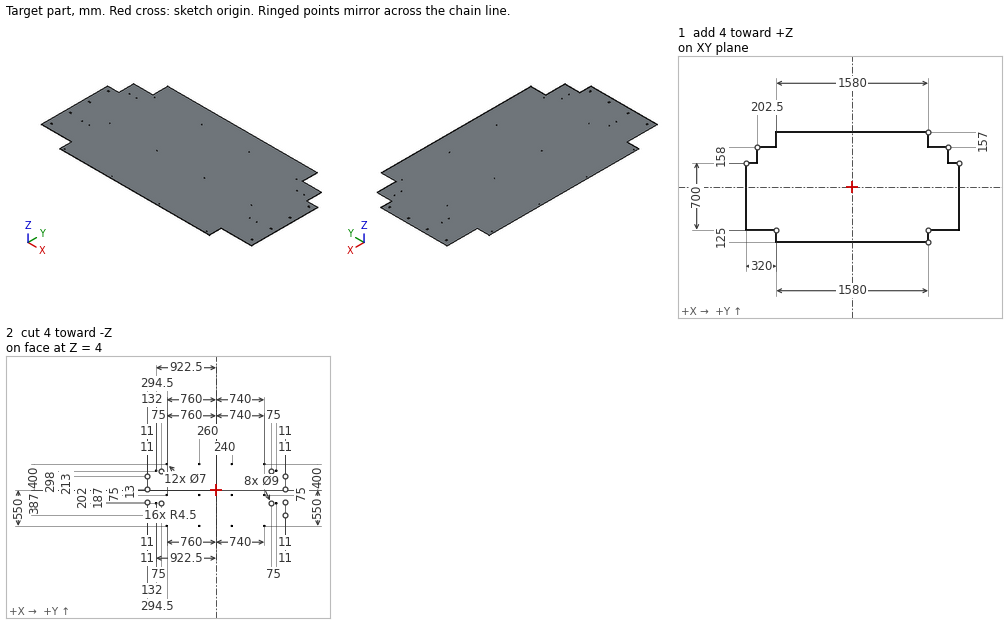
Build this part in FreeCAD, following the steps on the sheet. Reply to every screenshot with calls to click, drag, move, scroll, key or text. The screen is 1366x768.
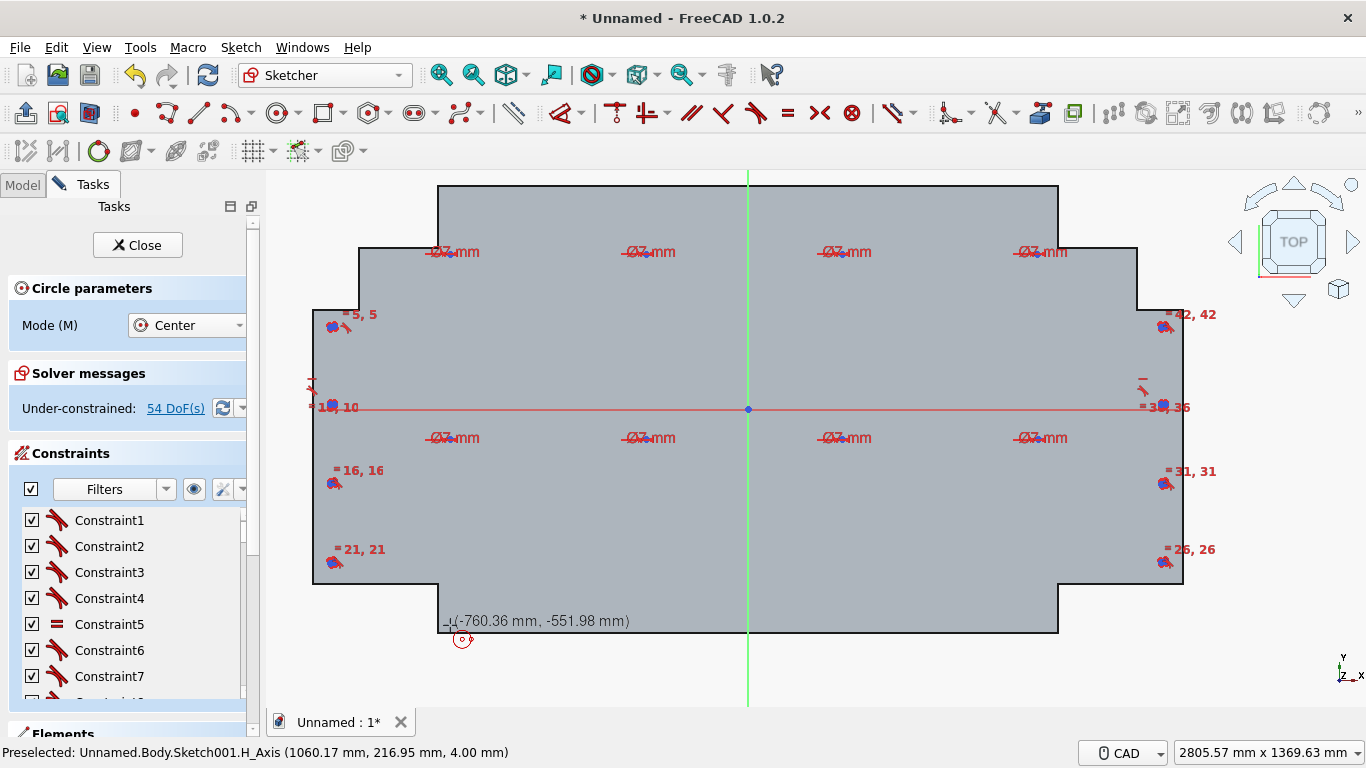
click(450, 625)
move(451, 624)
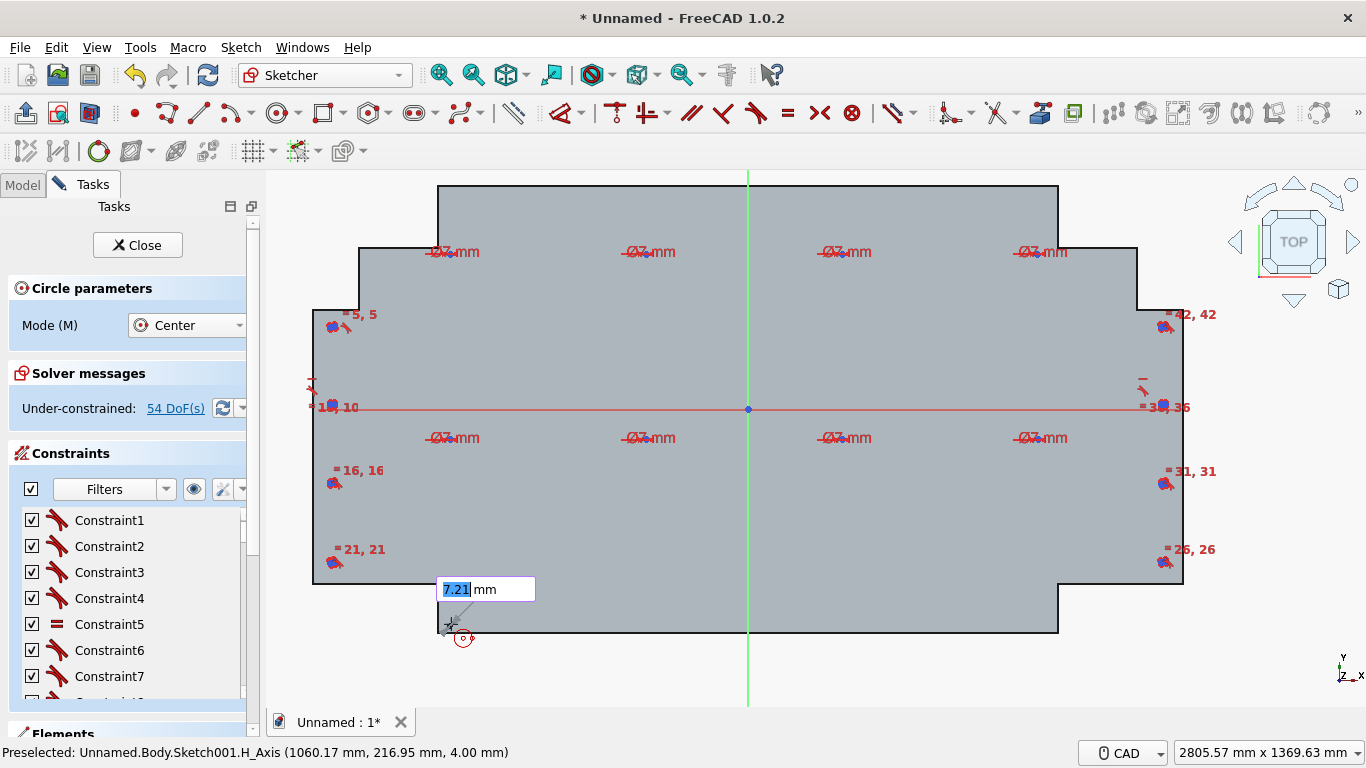
text(7)
key(Return)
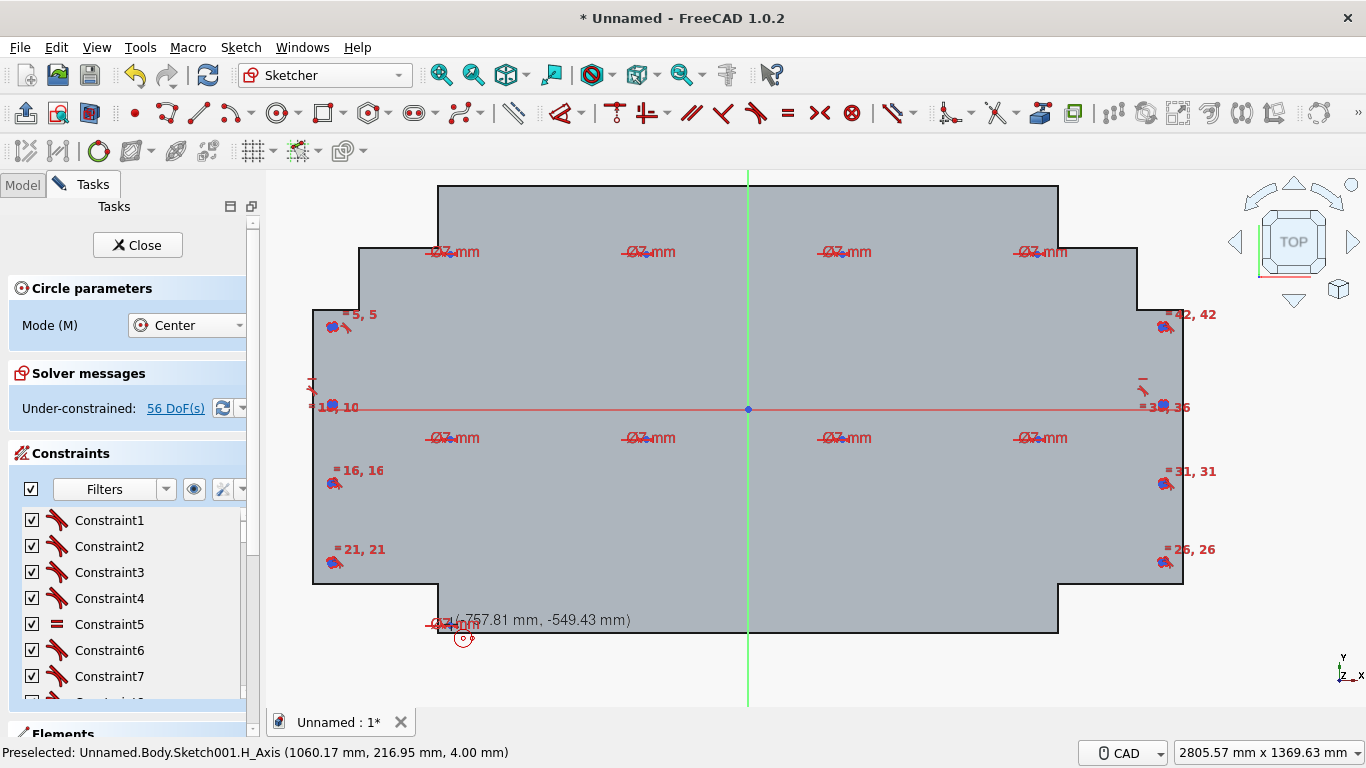
scroll(646, 625, up, 15)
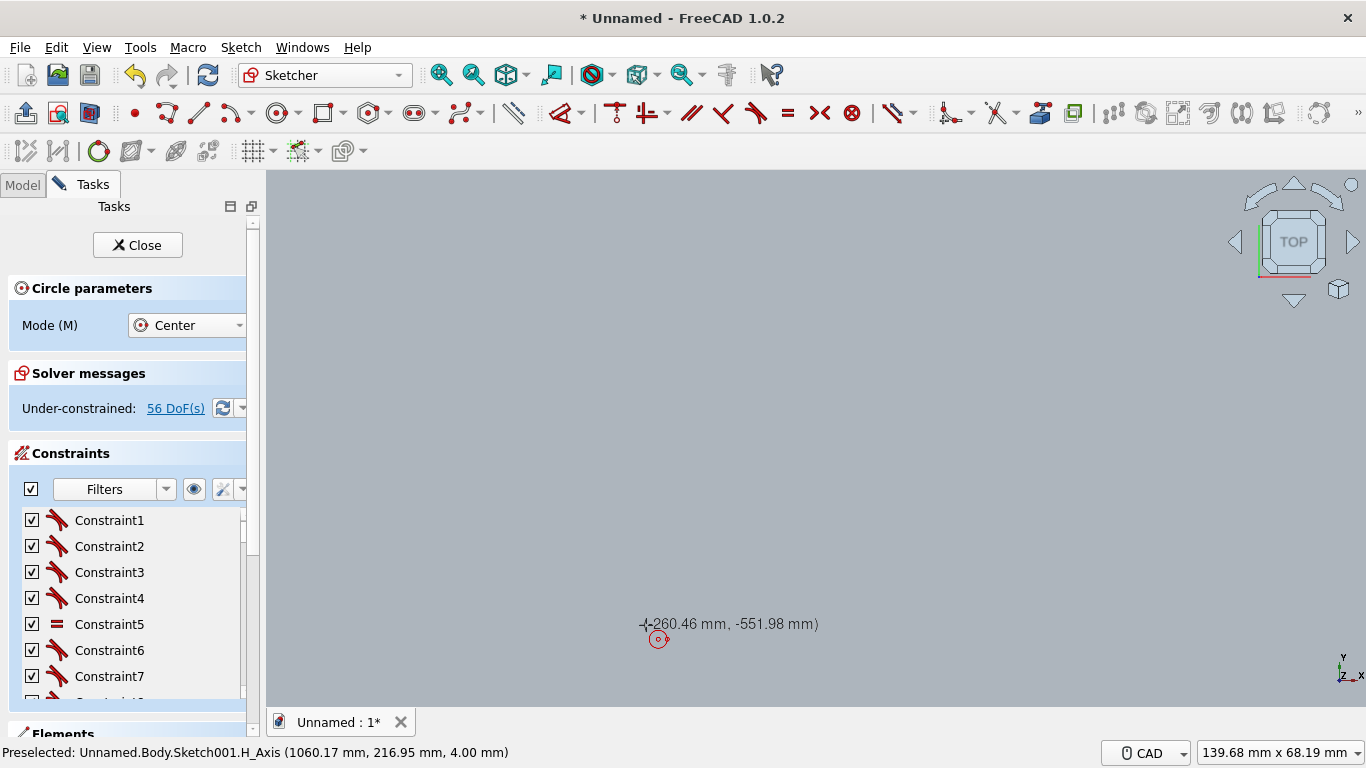
scroll(646, 625, down, 15)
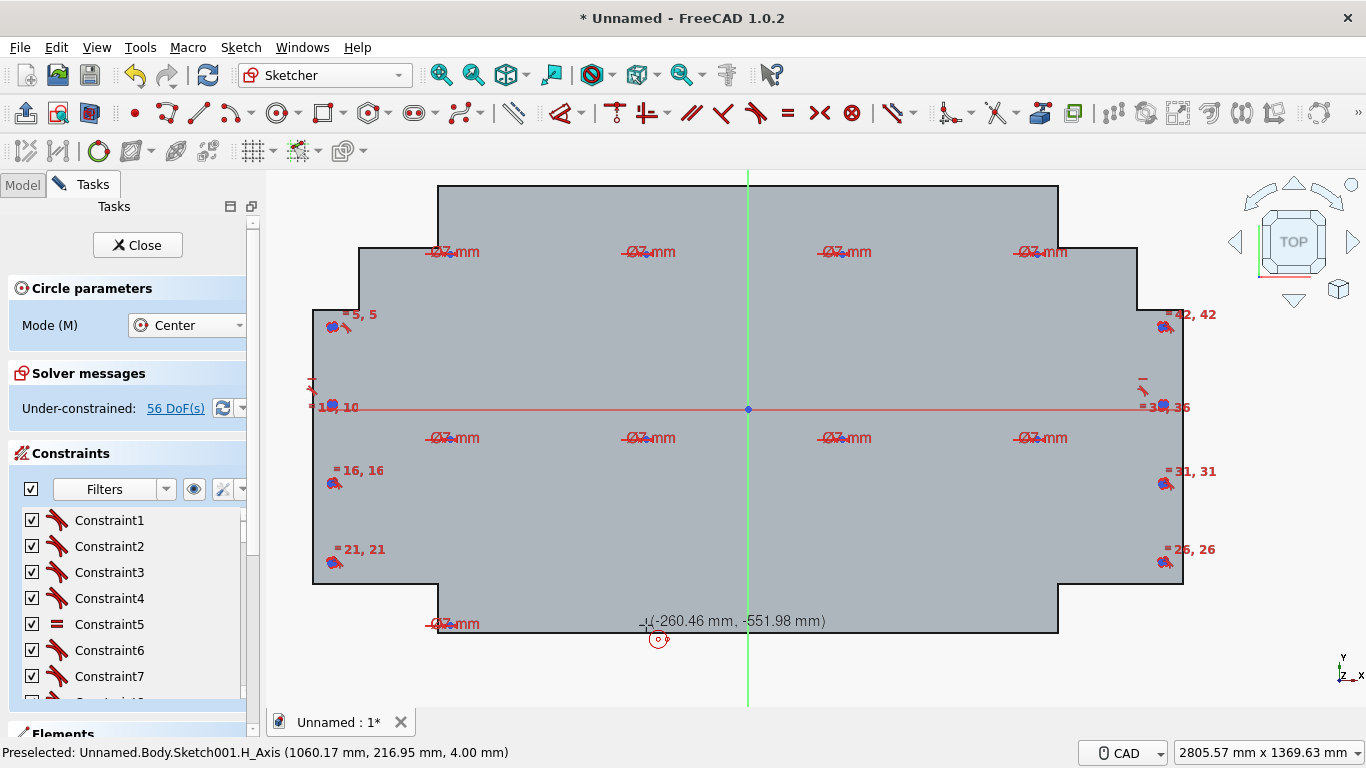
click(646, 625)
move(647, 624)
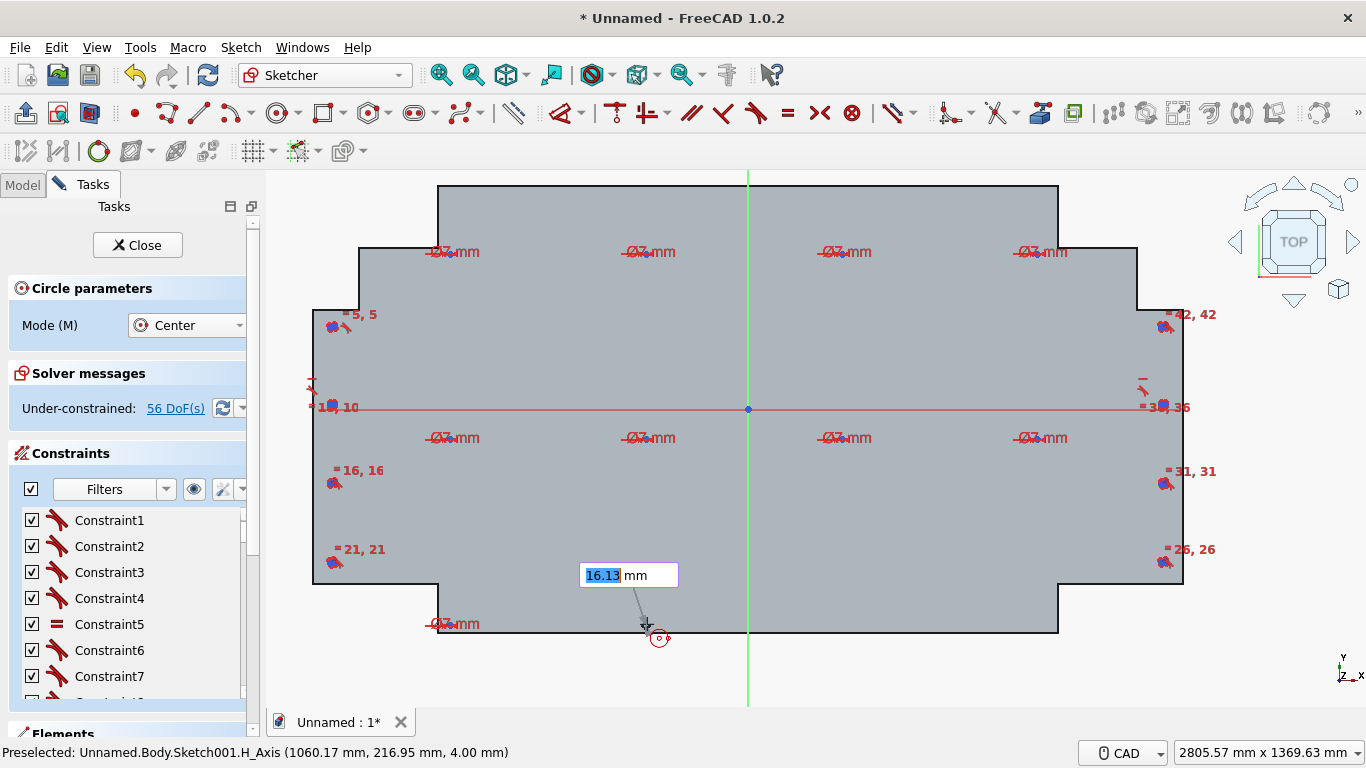
text(7)
key(Return)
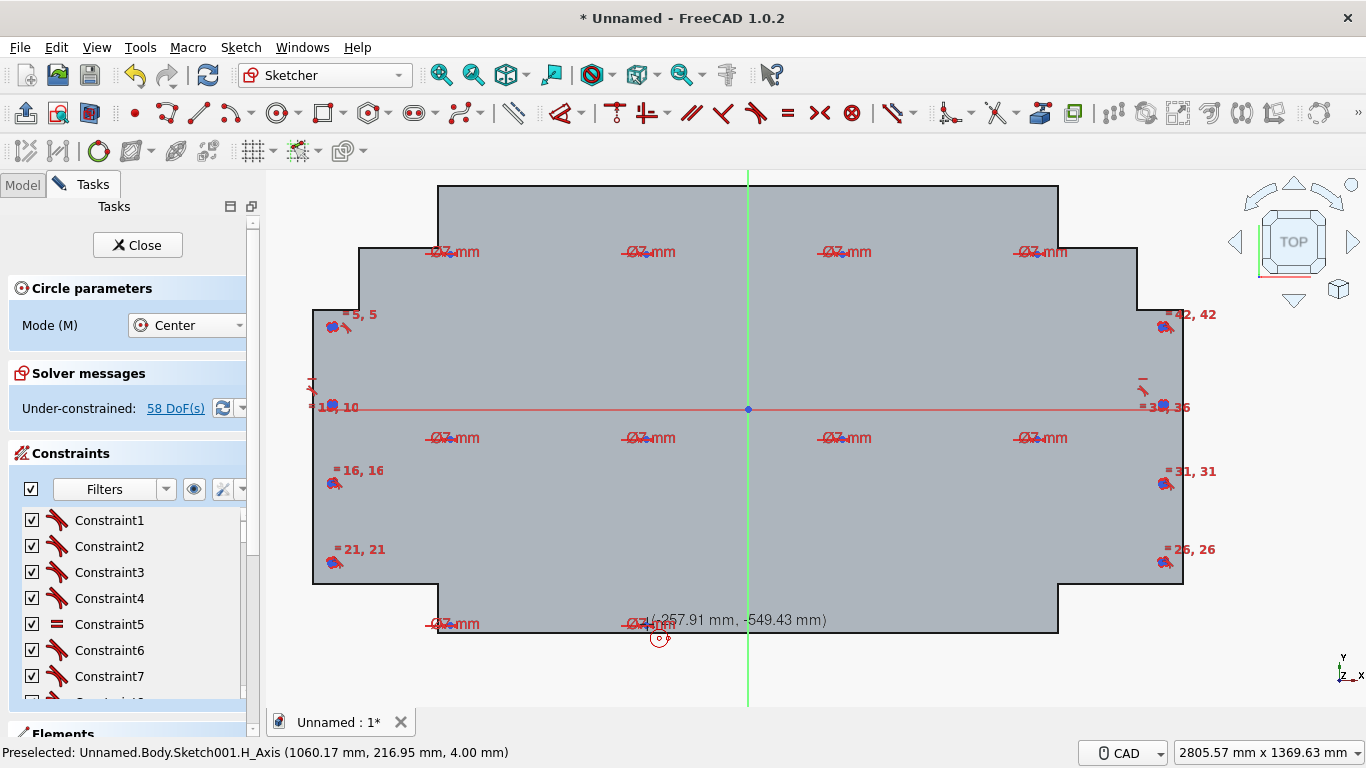
scroll(842, 625, up, 15)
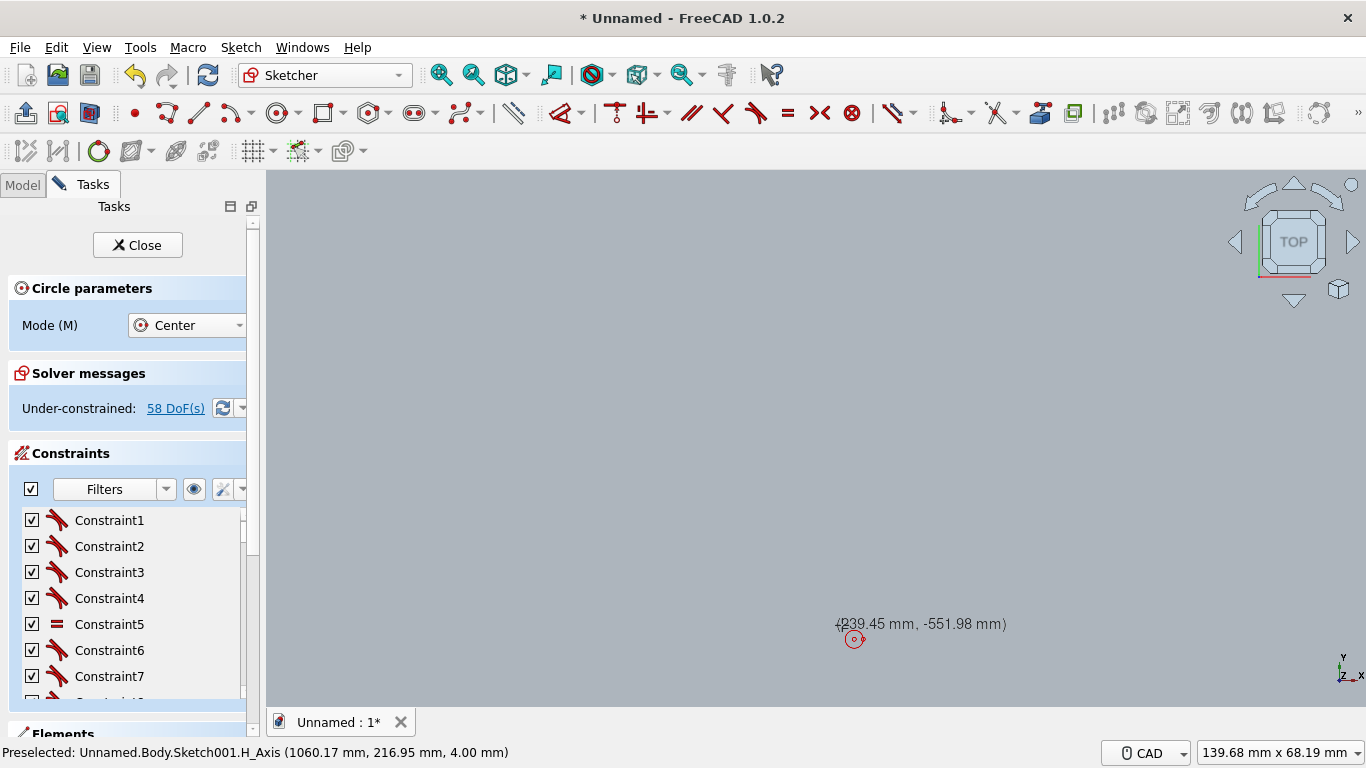
scroll(842, 625, down, 15)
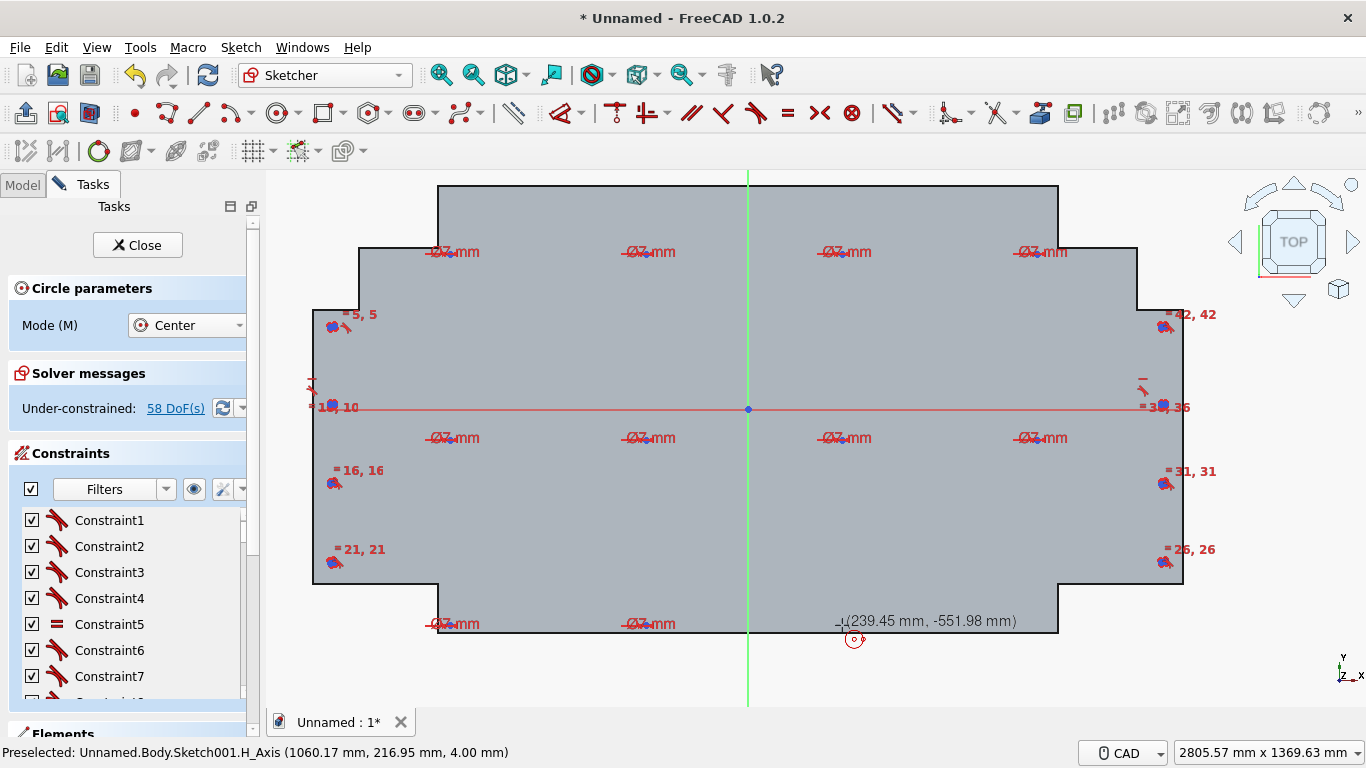
click(842, 625)
move(843, 624)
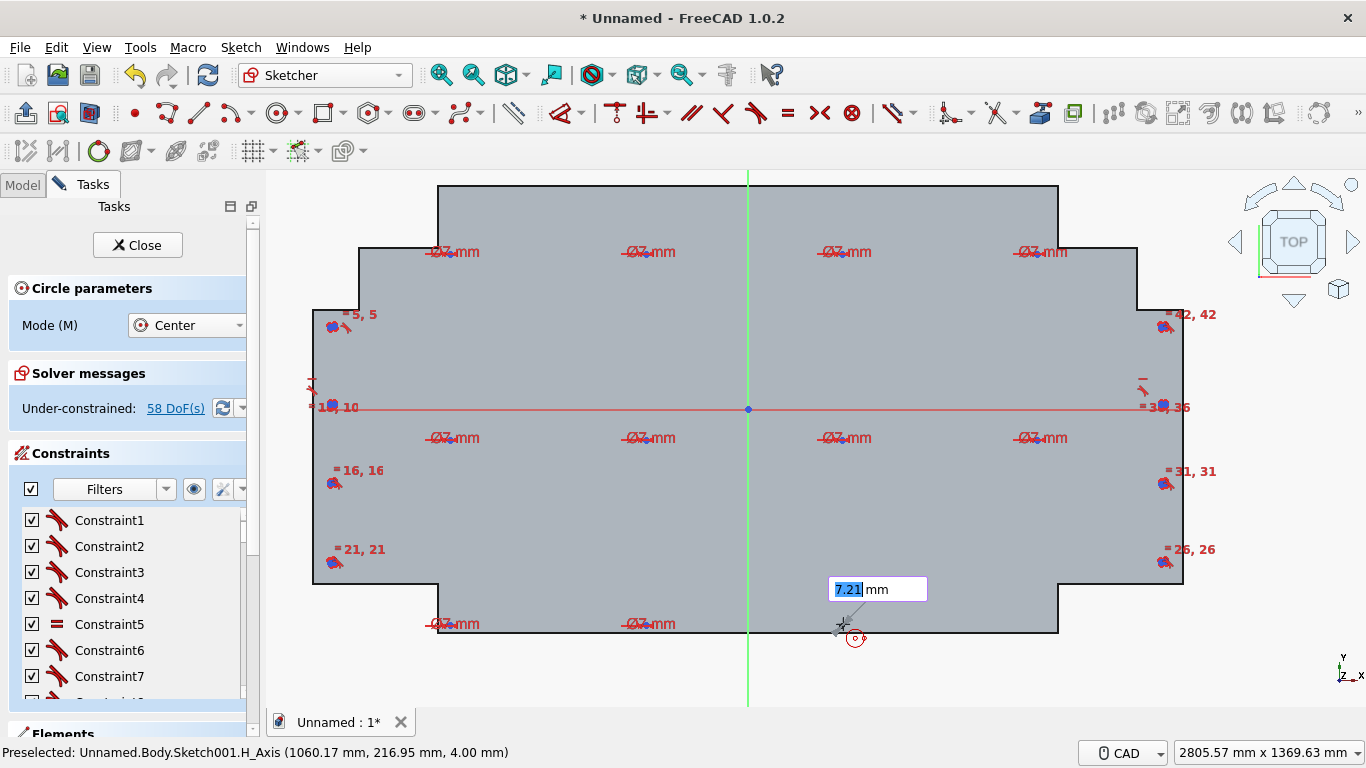
text(7)
key(Return)